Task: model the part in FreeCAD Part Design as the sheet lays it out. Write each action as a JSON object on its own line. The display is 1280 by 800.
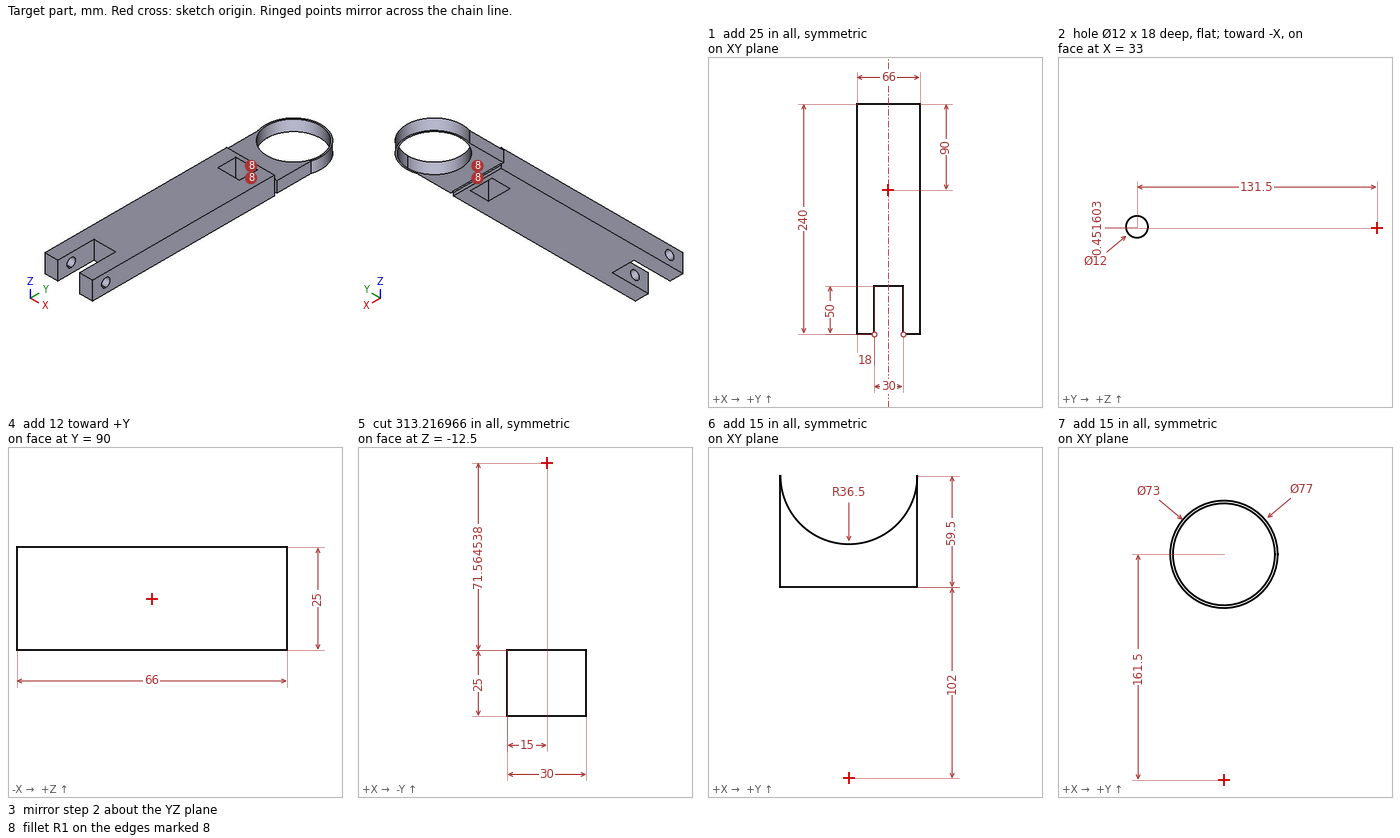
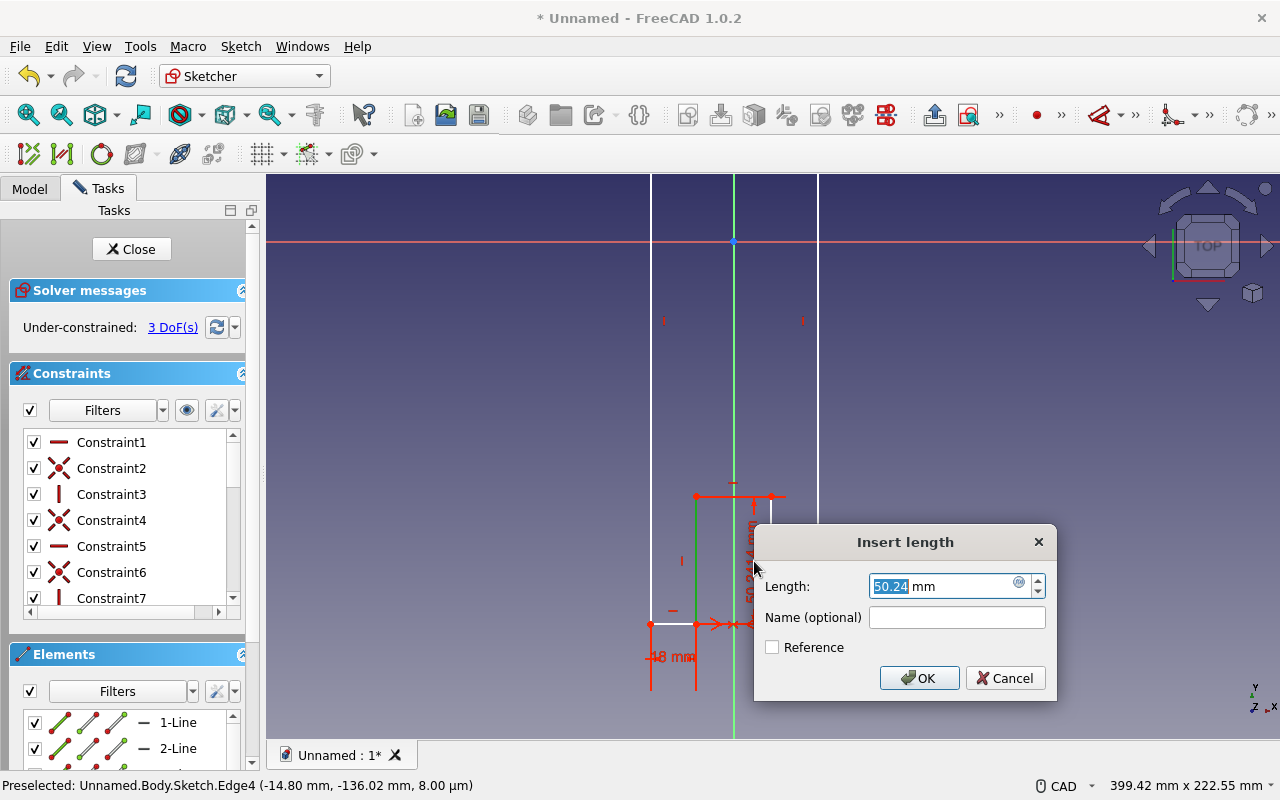
{"action": "type", "text": "50"}
{"action": "key", "text": "Return"}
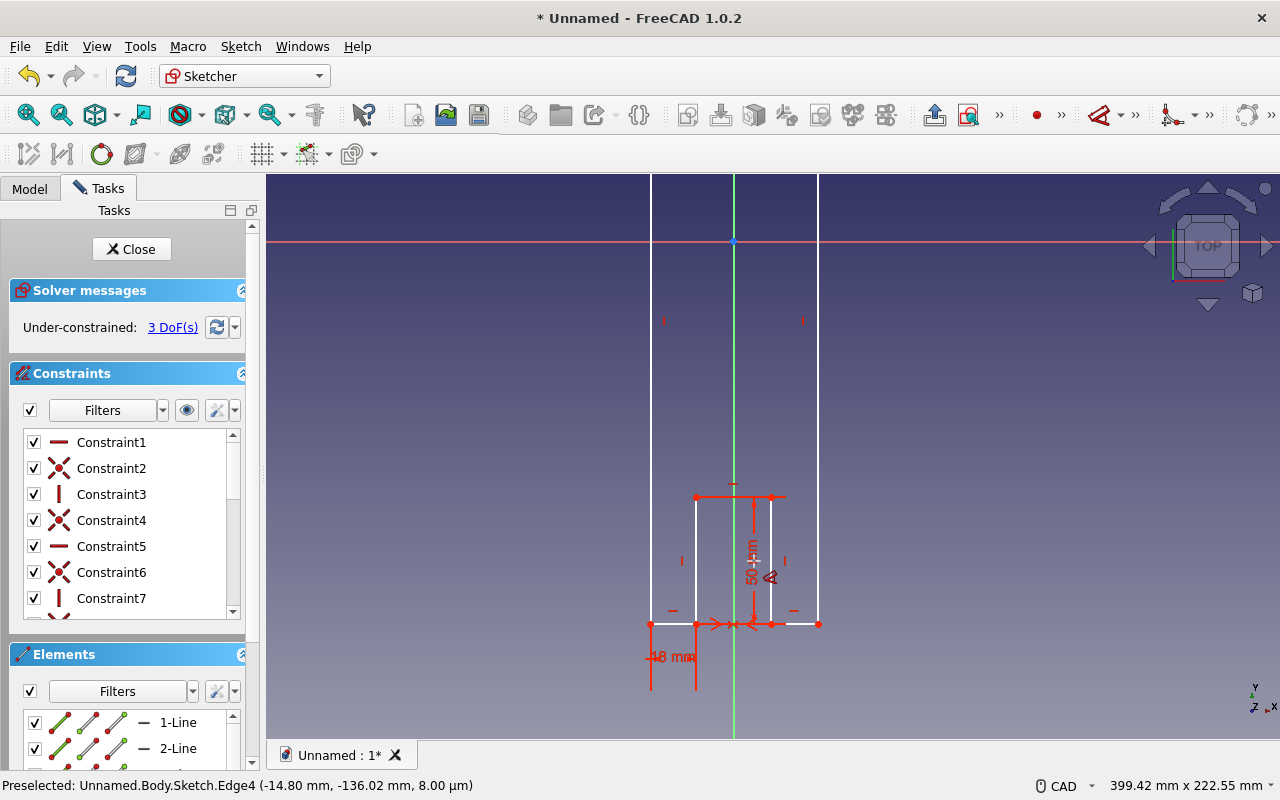
{"action": "left_click", "coordinate": [719, 497]}
{"action": "left_click", "coordinate": [717, 531]}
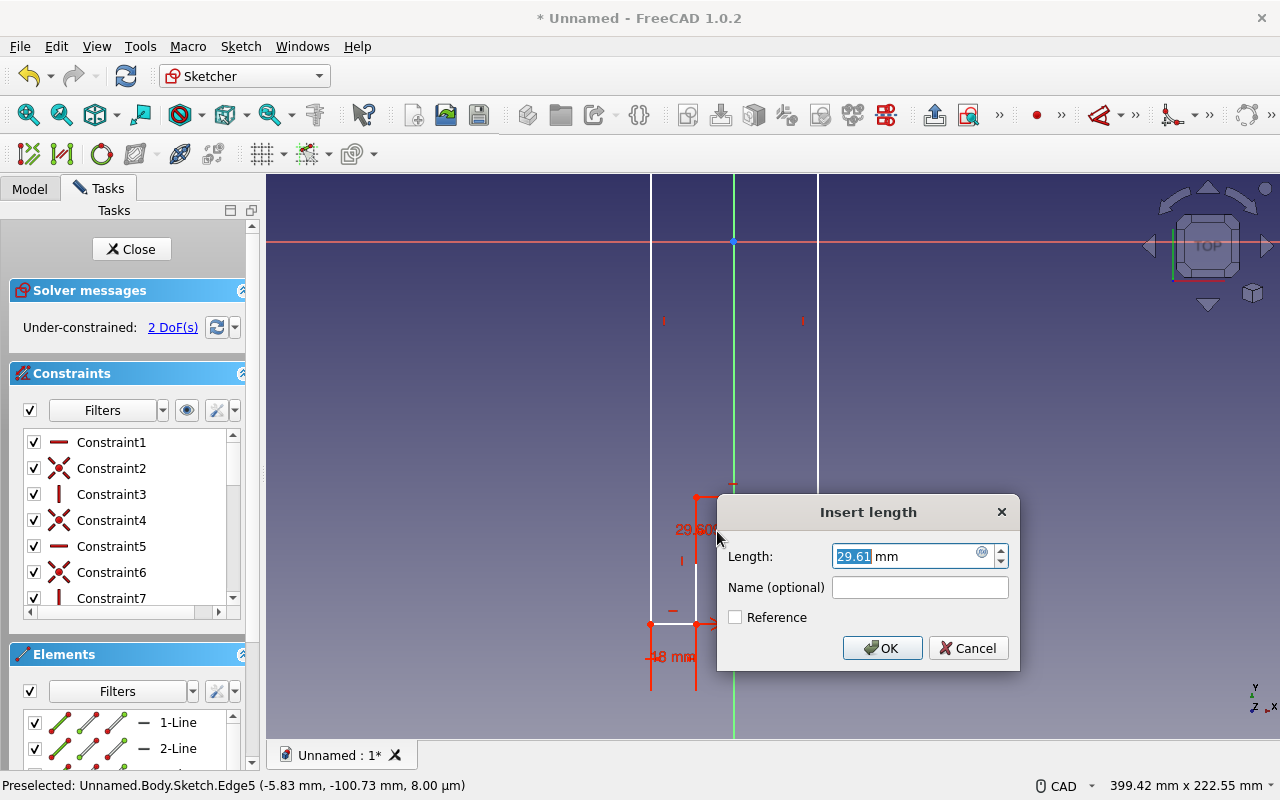
{"action": "type", "text": "30"}
{"action": "key", "text": "Return"}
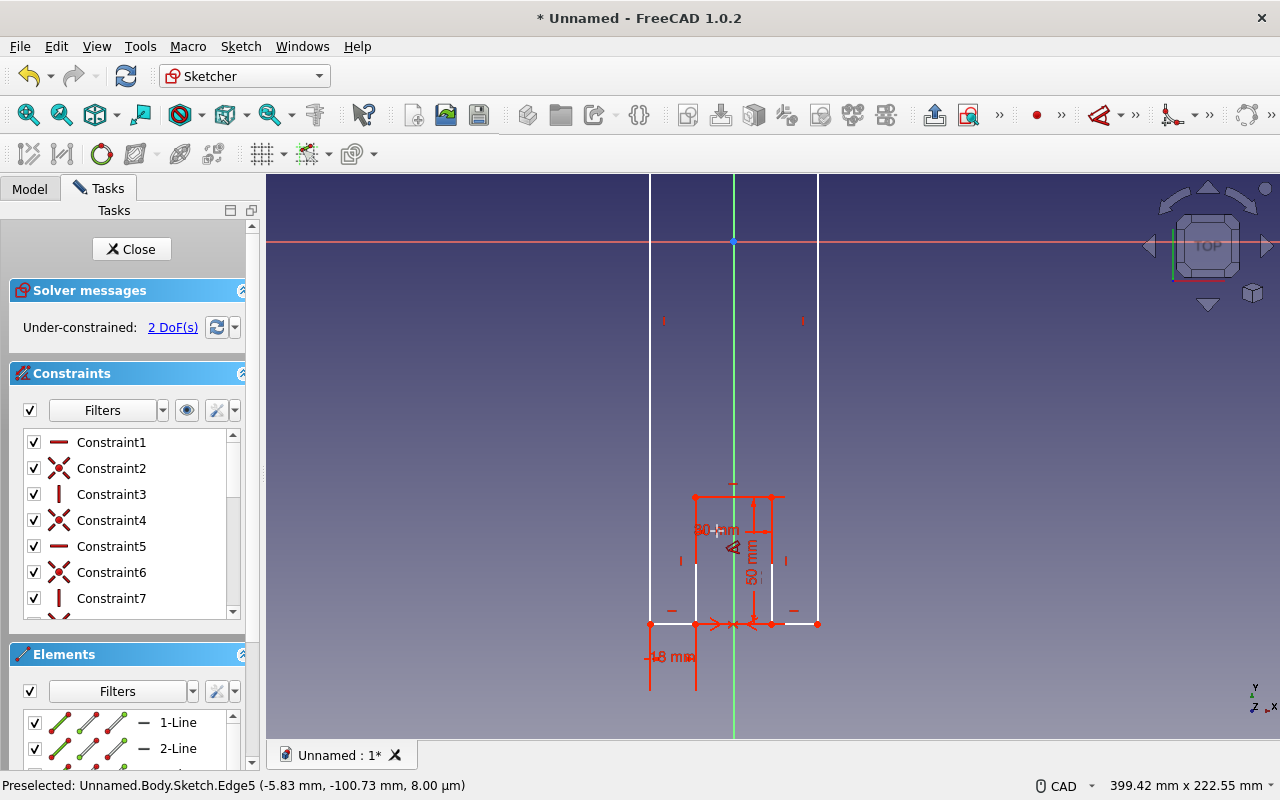
{"action": "left_click", "coordinate": [650, 442]}
{"action": "left_click", "coordinate": [616, 413]}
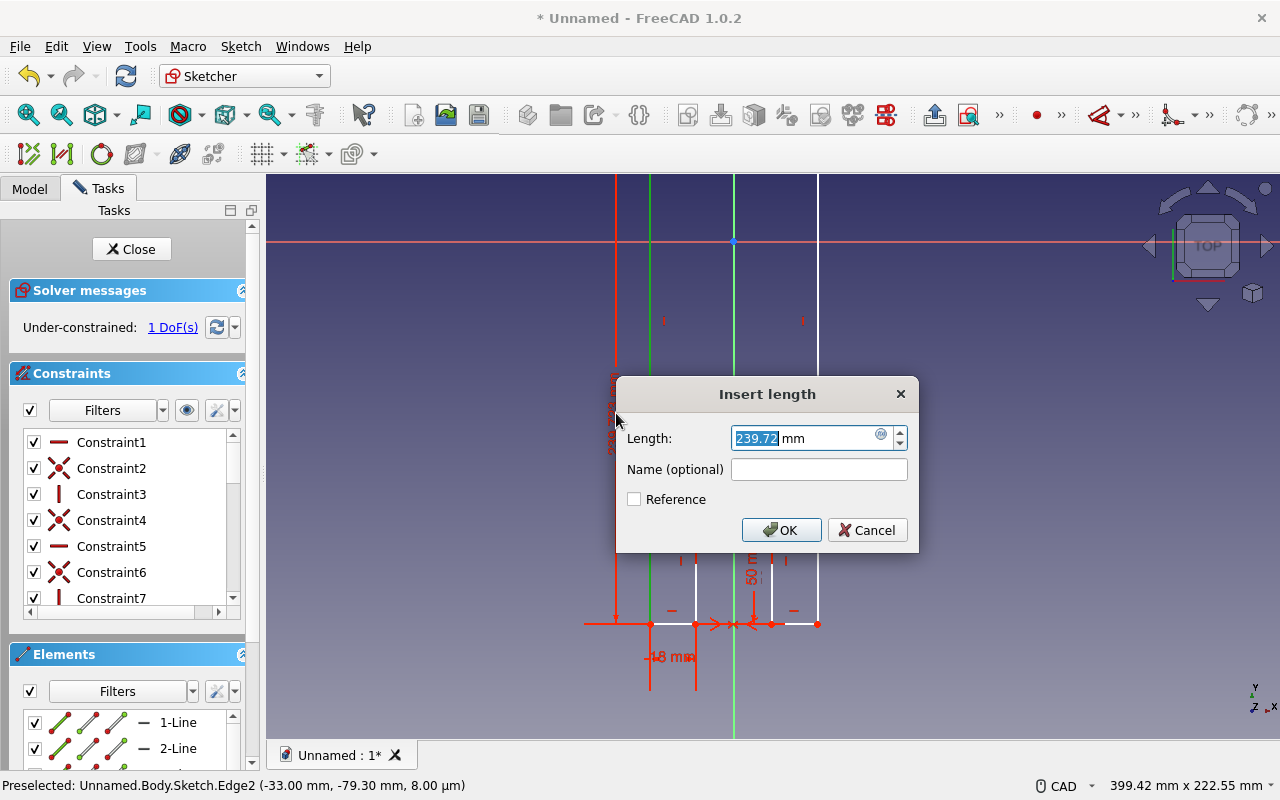
{"action": "type", "text": "240"}
{"action": "key", "text": "Return"}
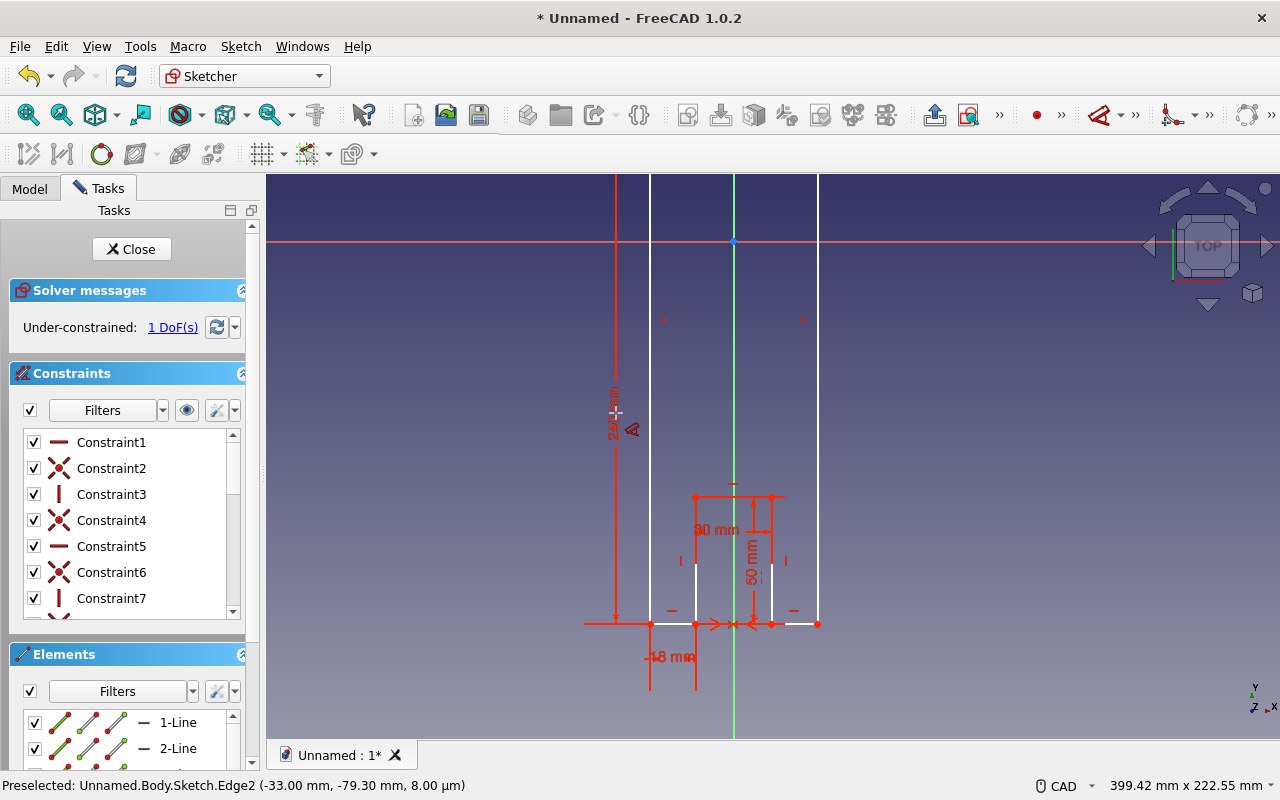
{"action": "scroll", "coordinate": [669, 625], "scroll_direction": "down", "scroll_amount": 3}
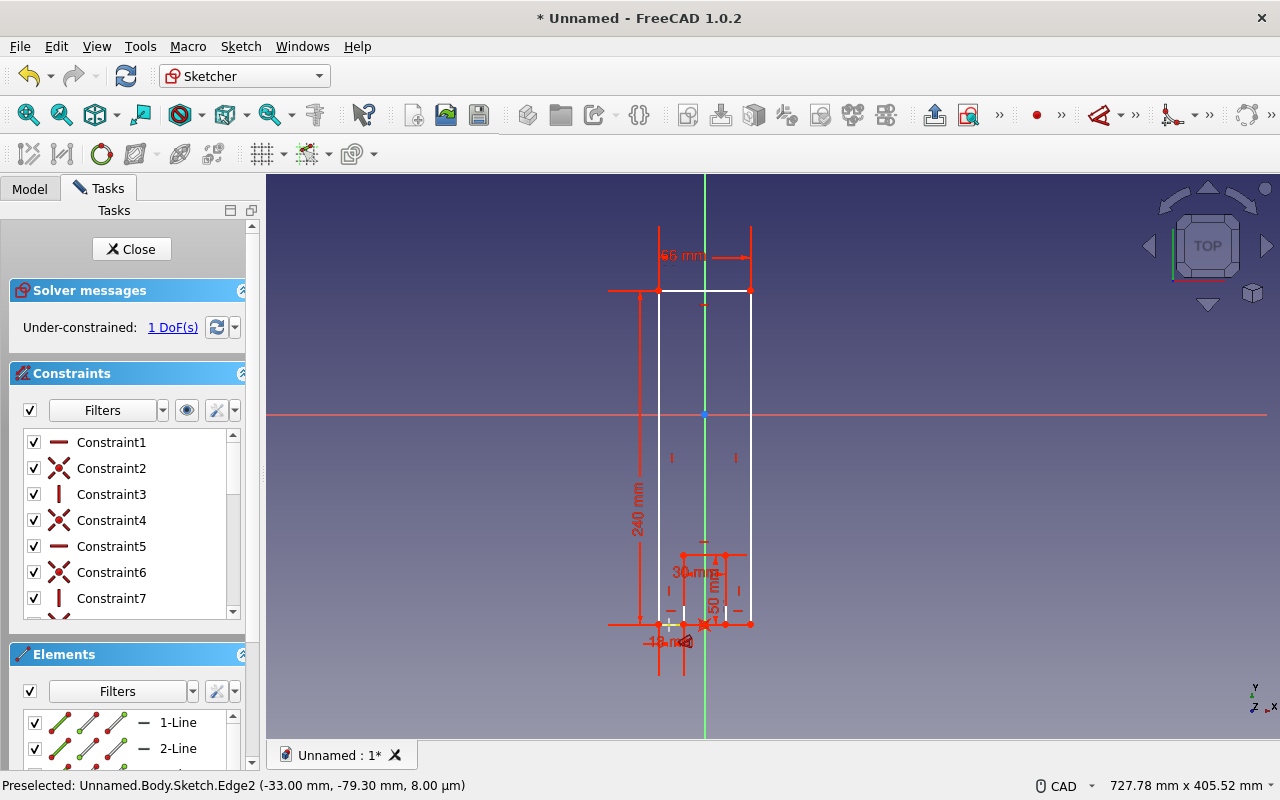
{"action": "left_click", "coordinate": [751, 291]}
{"action": "left_click", "coordinate": [785, 353]}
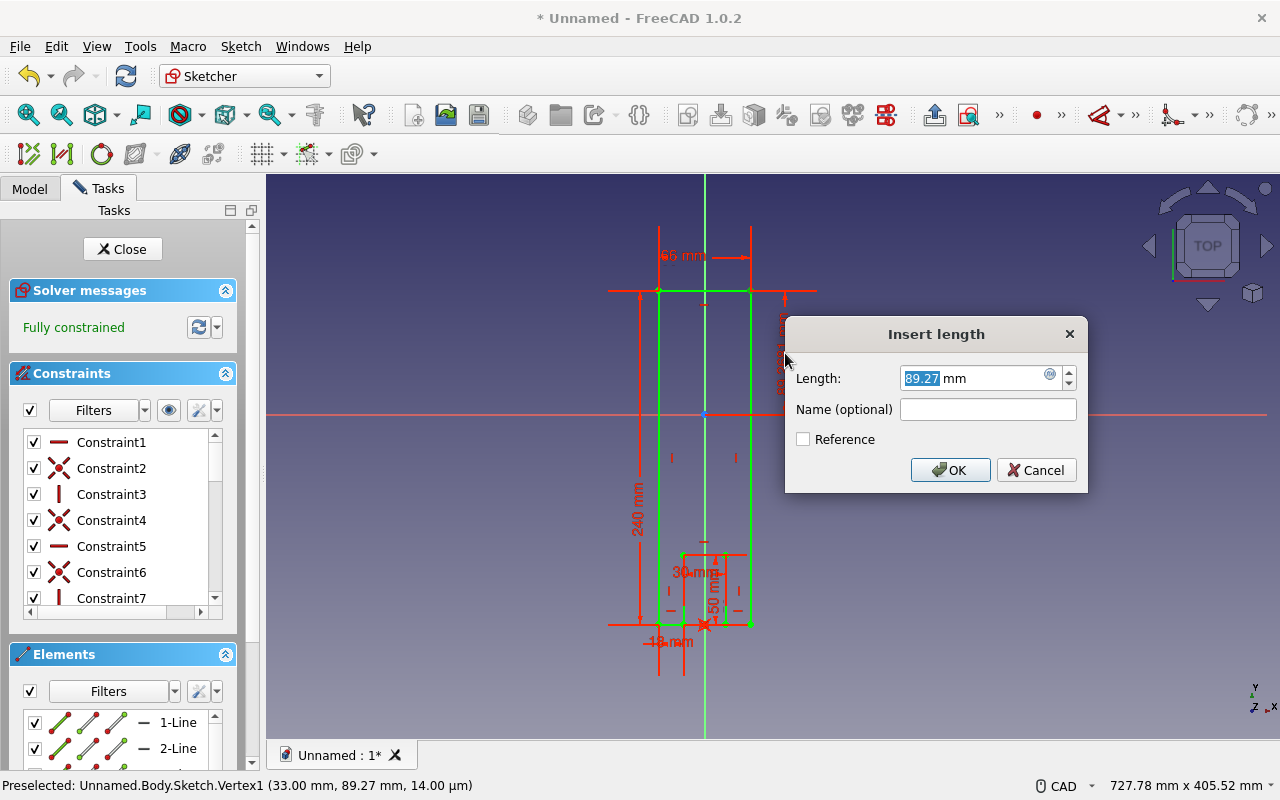
{"action": "type", "text": "90"}
{"action": "key", "text": "Return"}
{"action": "key", "text": "Escape"}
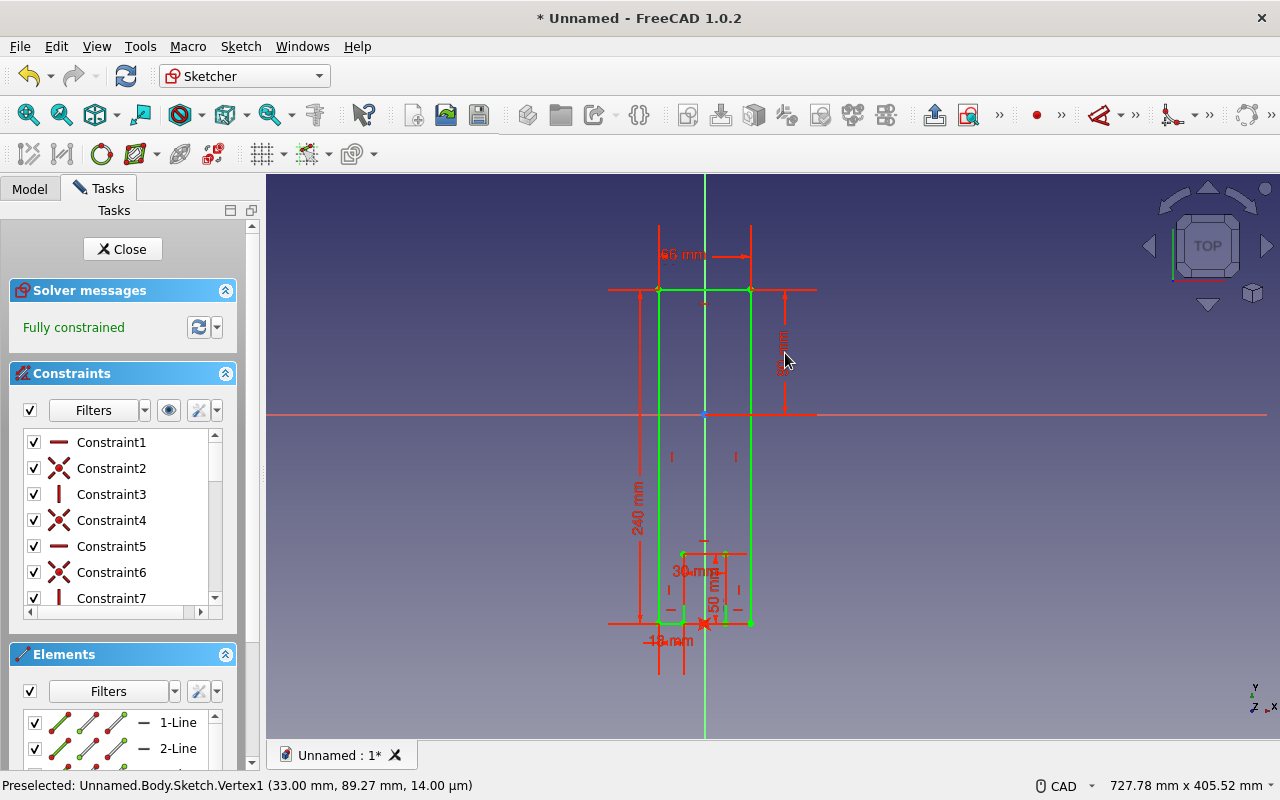
{"action": "left_click", "coordinate": [123, 249]}